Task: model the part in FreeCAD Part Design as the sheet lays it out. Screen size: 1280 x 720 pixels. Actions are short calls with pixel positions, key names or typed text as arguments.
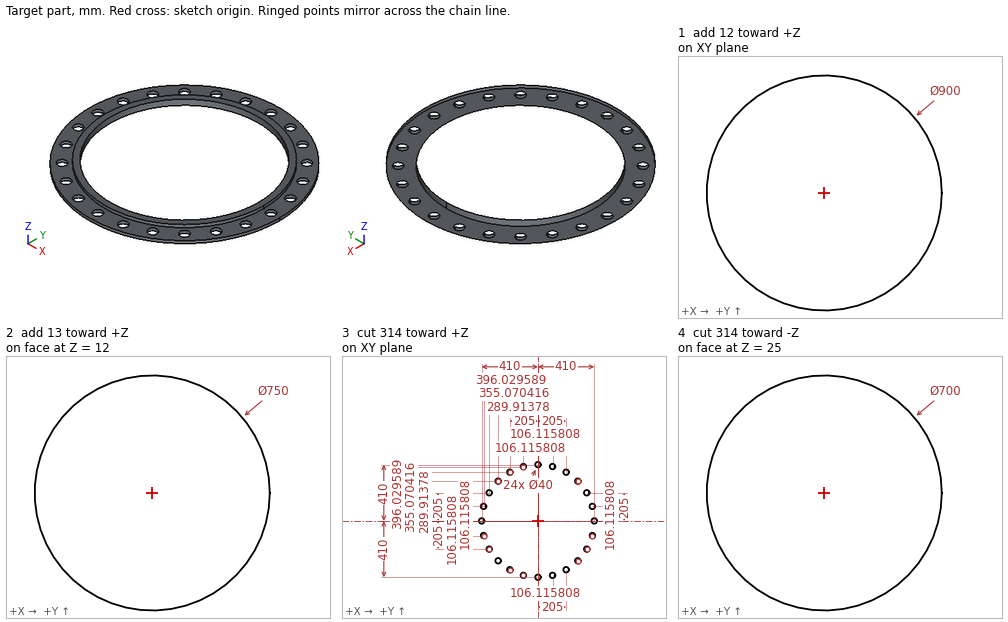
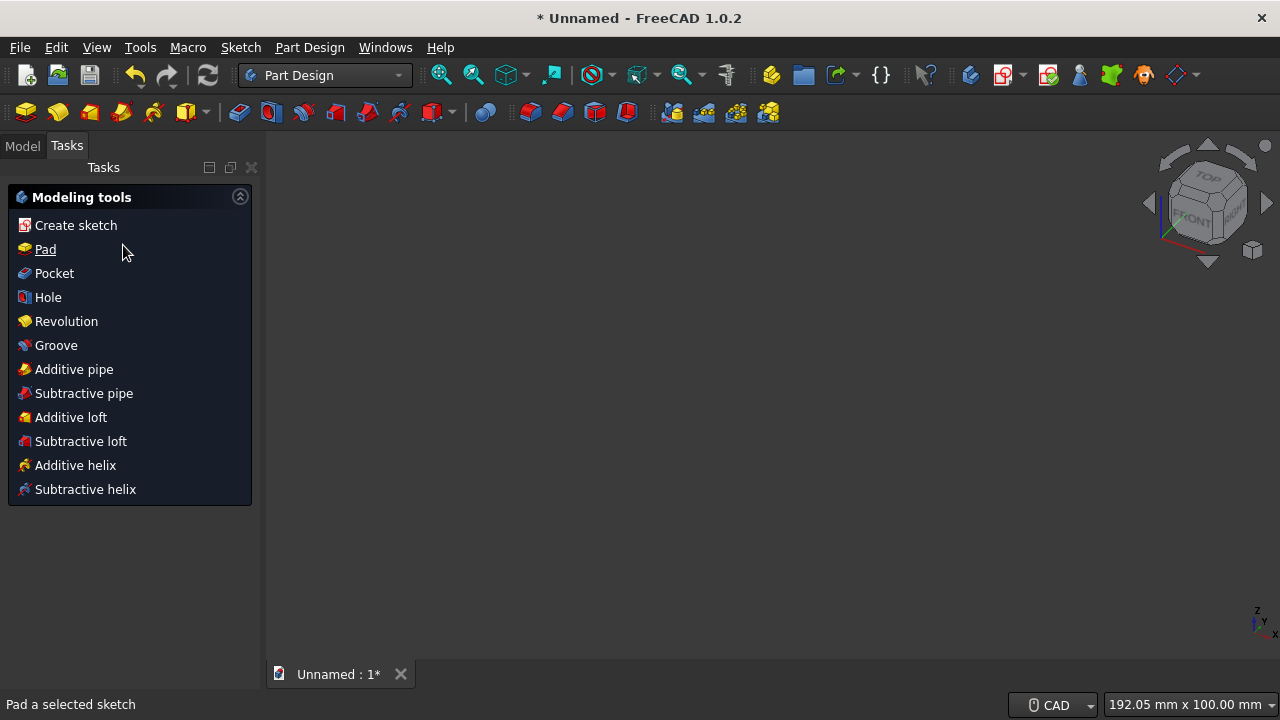
click(26, 112)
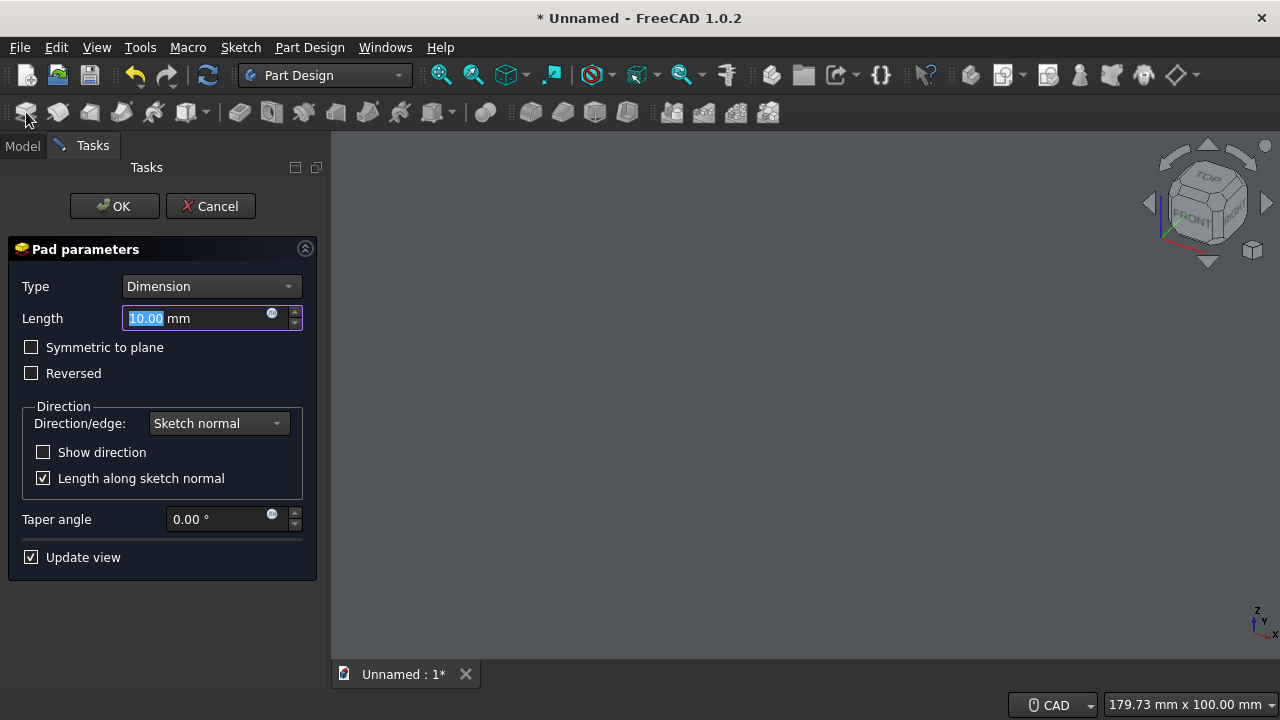
text(12)
key(Tab)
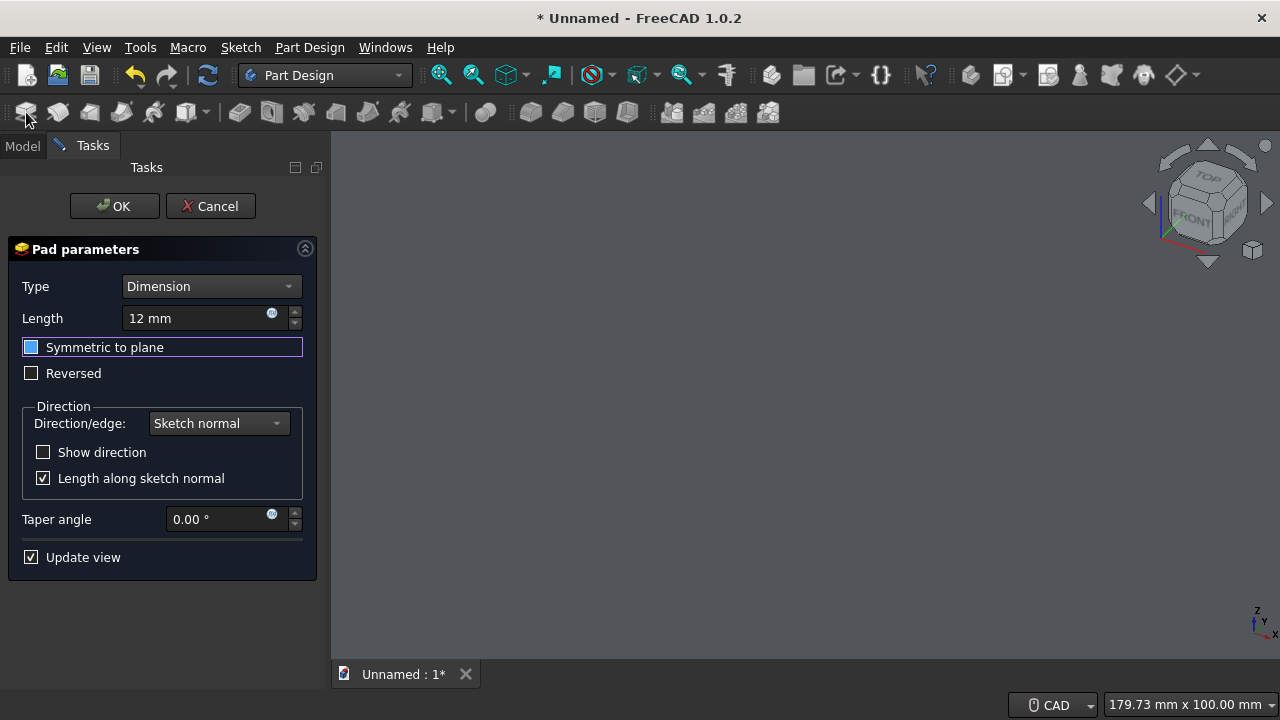
click(115, 206)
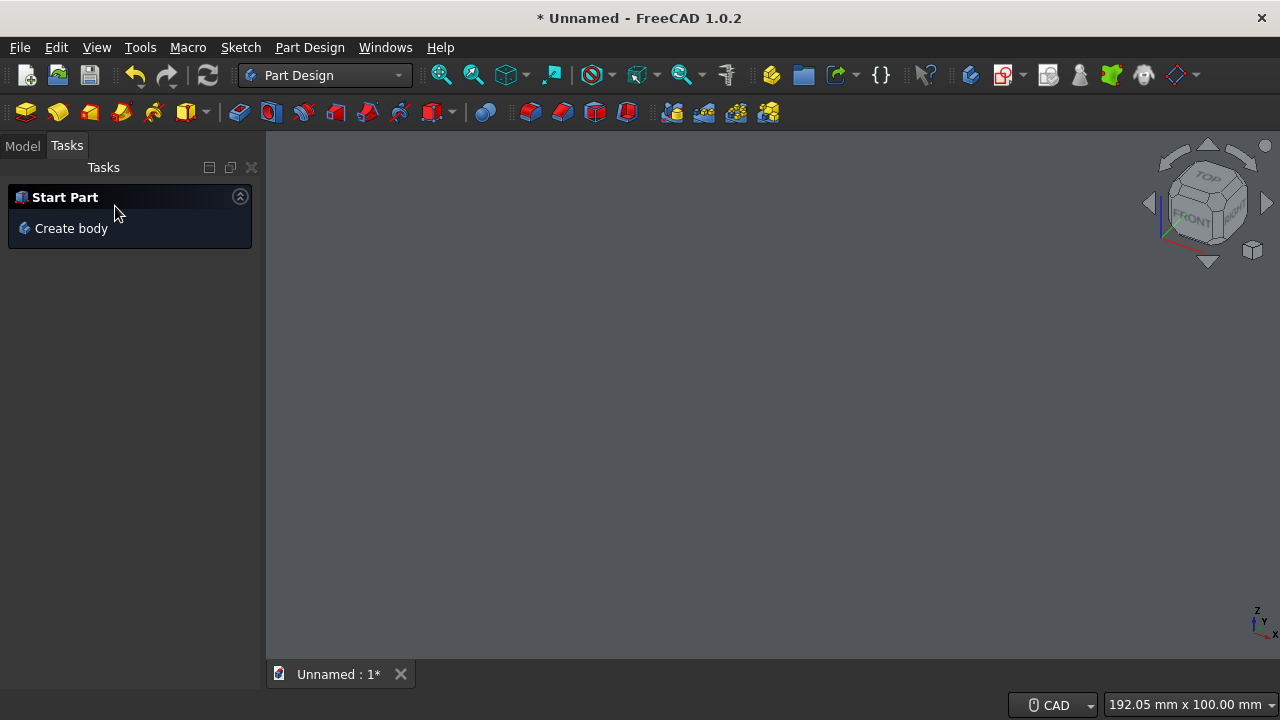
click(442, 76)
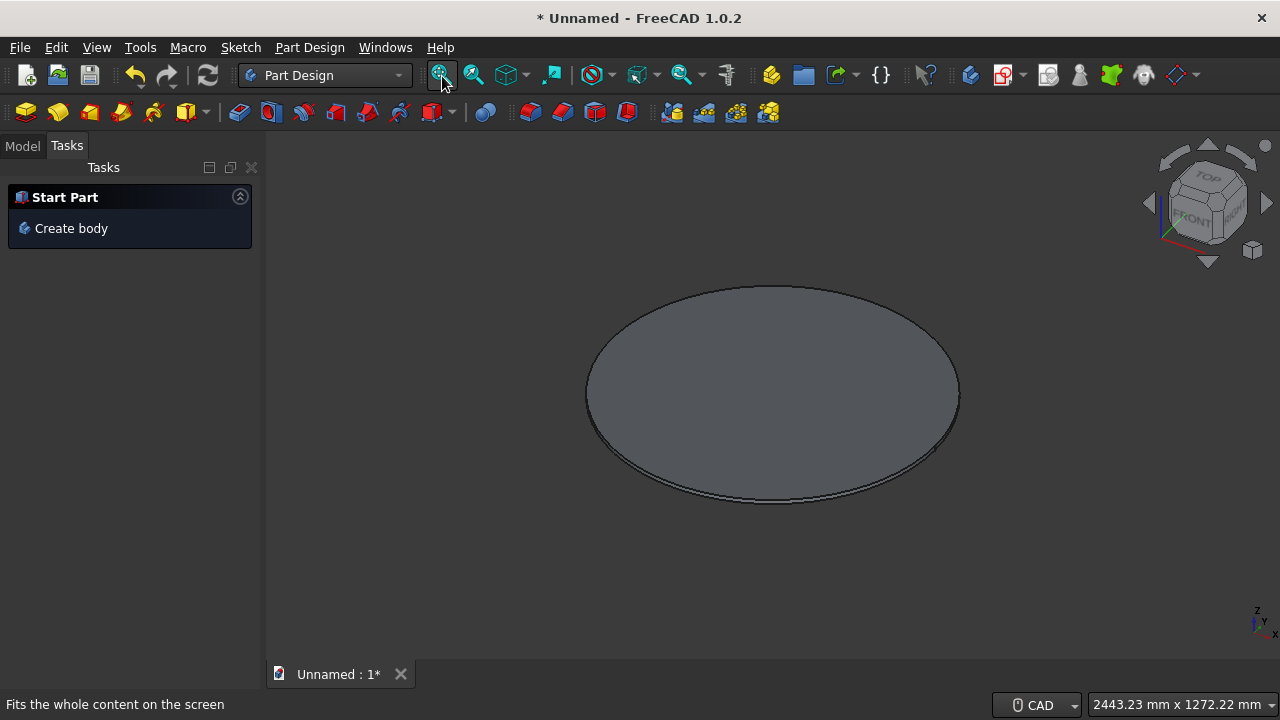
click(773, 392)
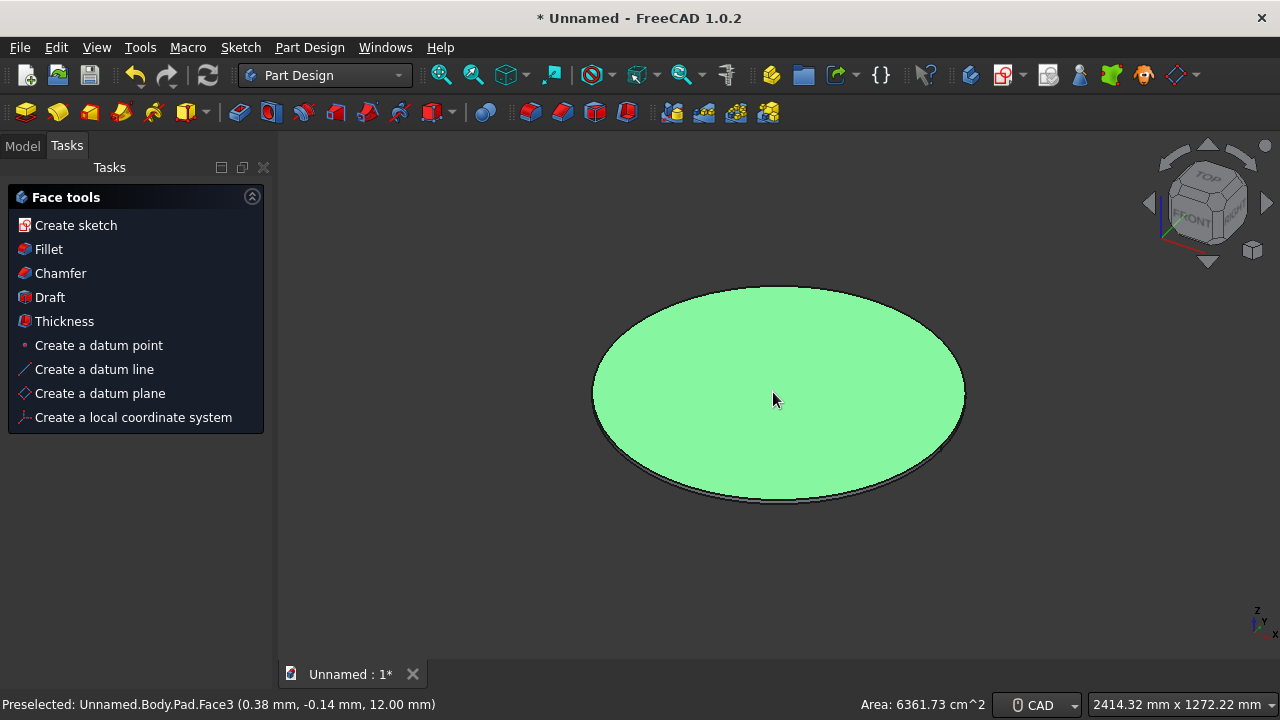
click(1004, 76)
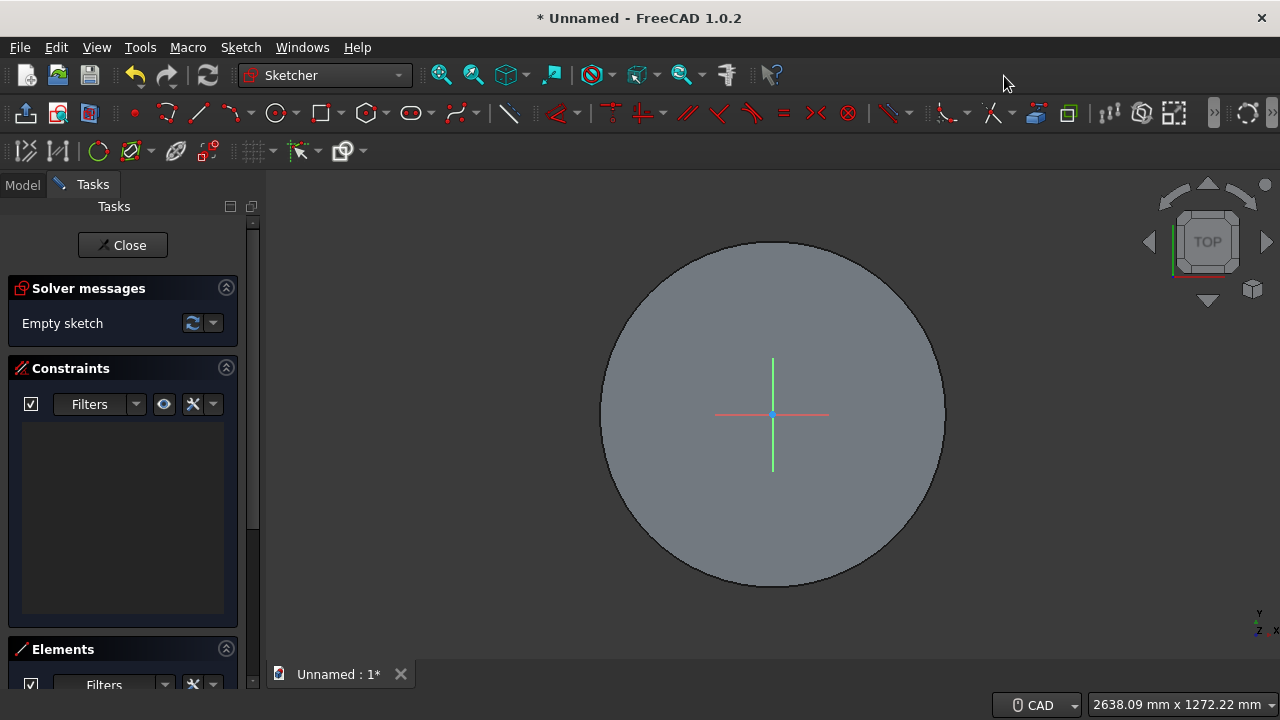
click(276, 114)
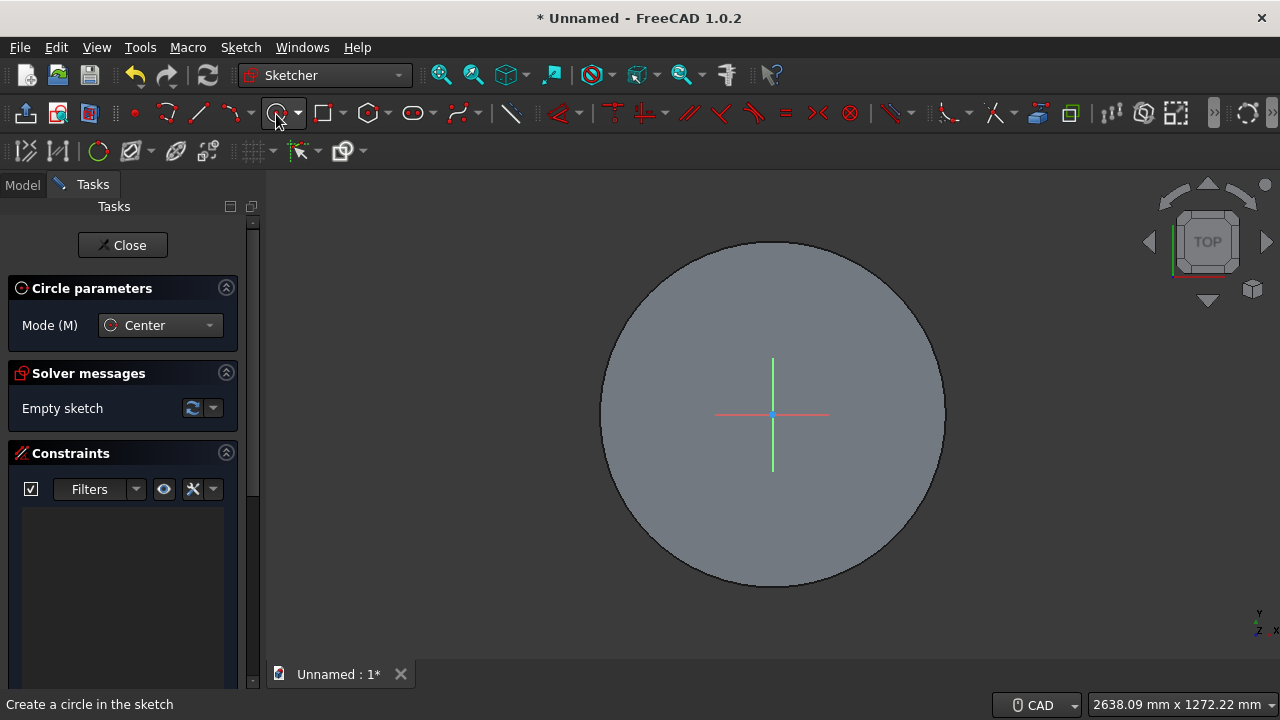
click(773, 414)
click(875, 313)
key(Escape)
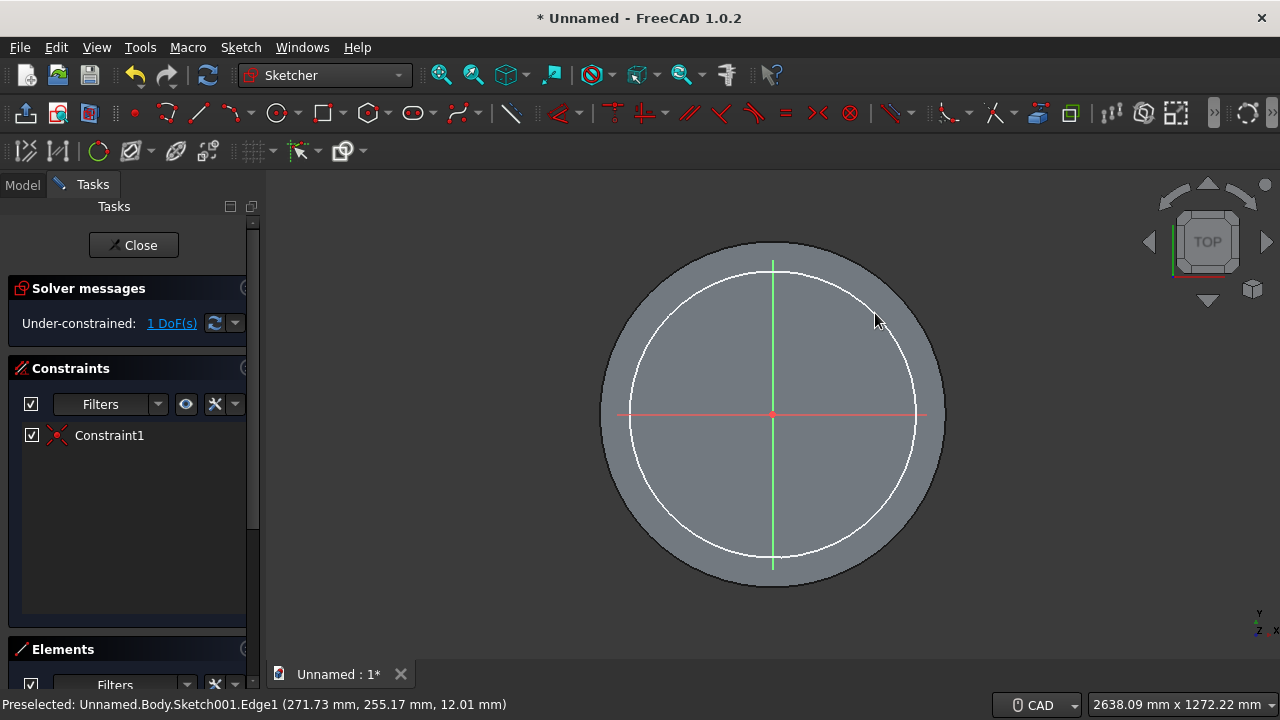
click(558, 114)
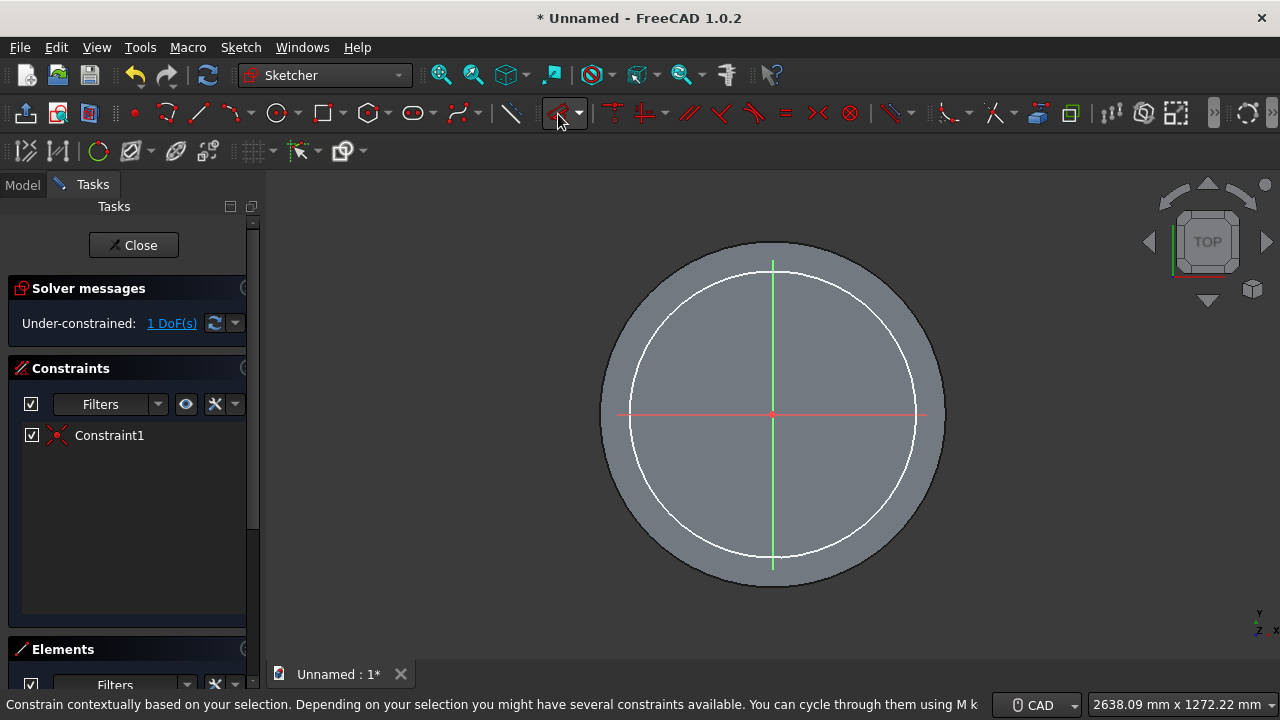
click(874, 313)
click(897, 290)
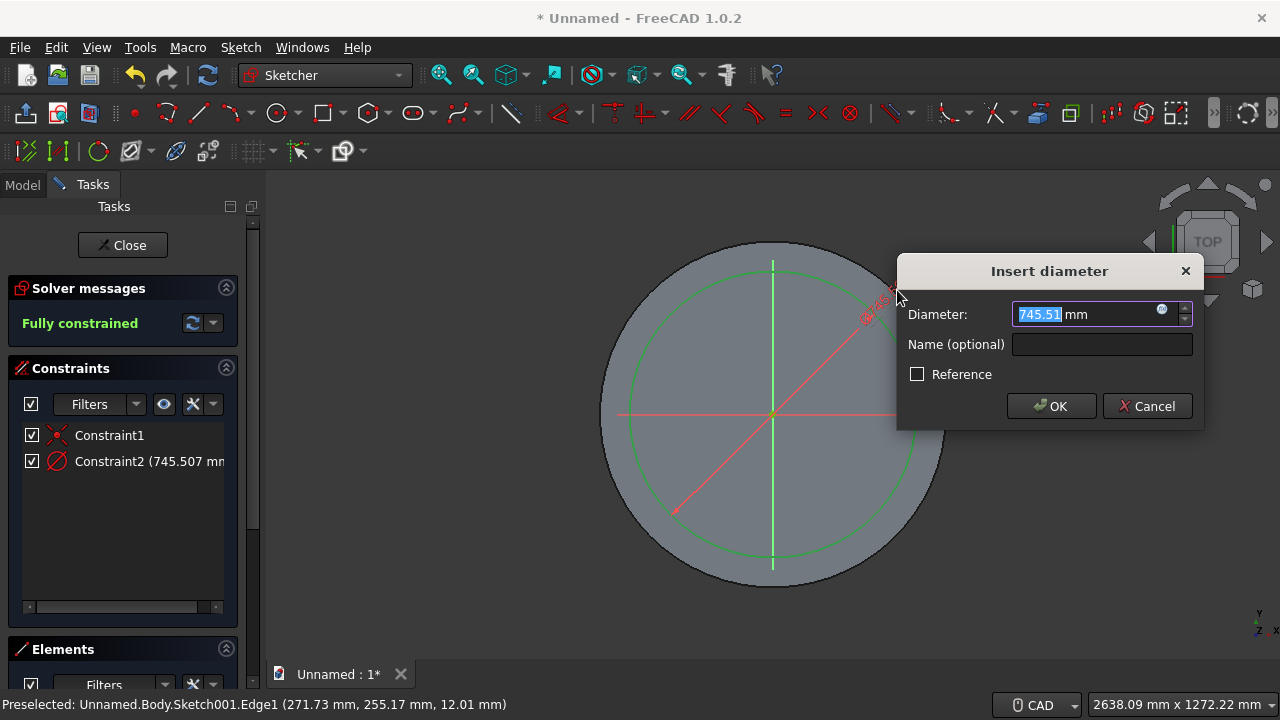
text(750)
key(Return)
key(Escape)